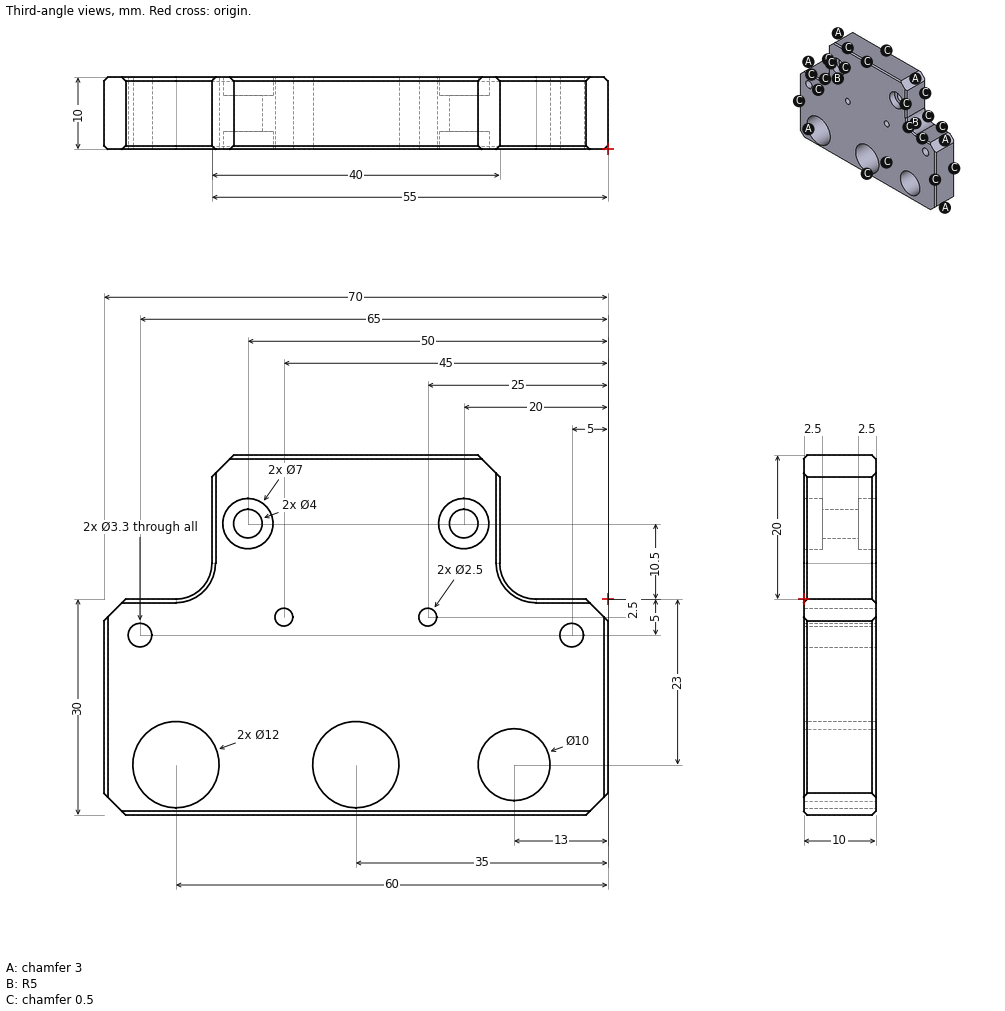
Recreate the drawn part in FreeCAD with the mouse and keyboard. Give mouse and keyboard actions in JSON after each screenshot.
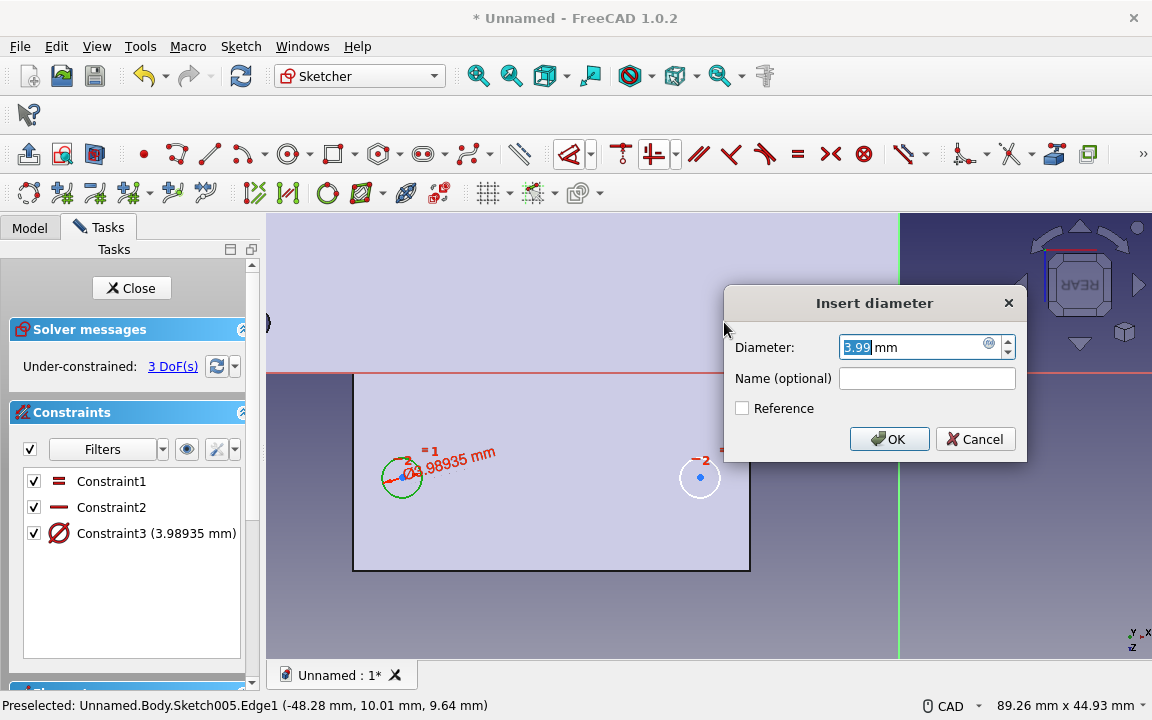
{"action": "type", "text": "4"}
{"action": "key", "text": "Return"}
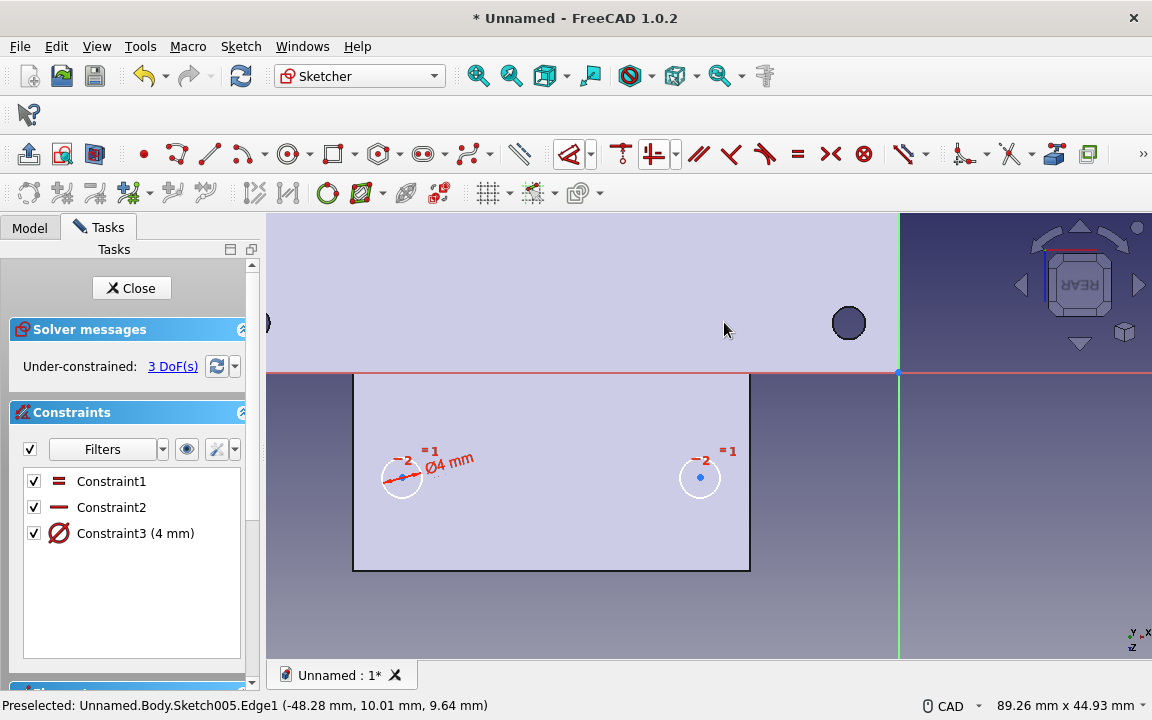
{"action": "left_click", "coordinate": [402, 478]}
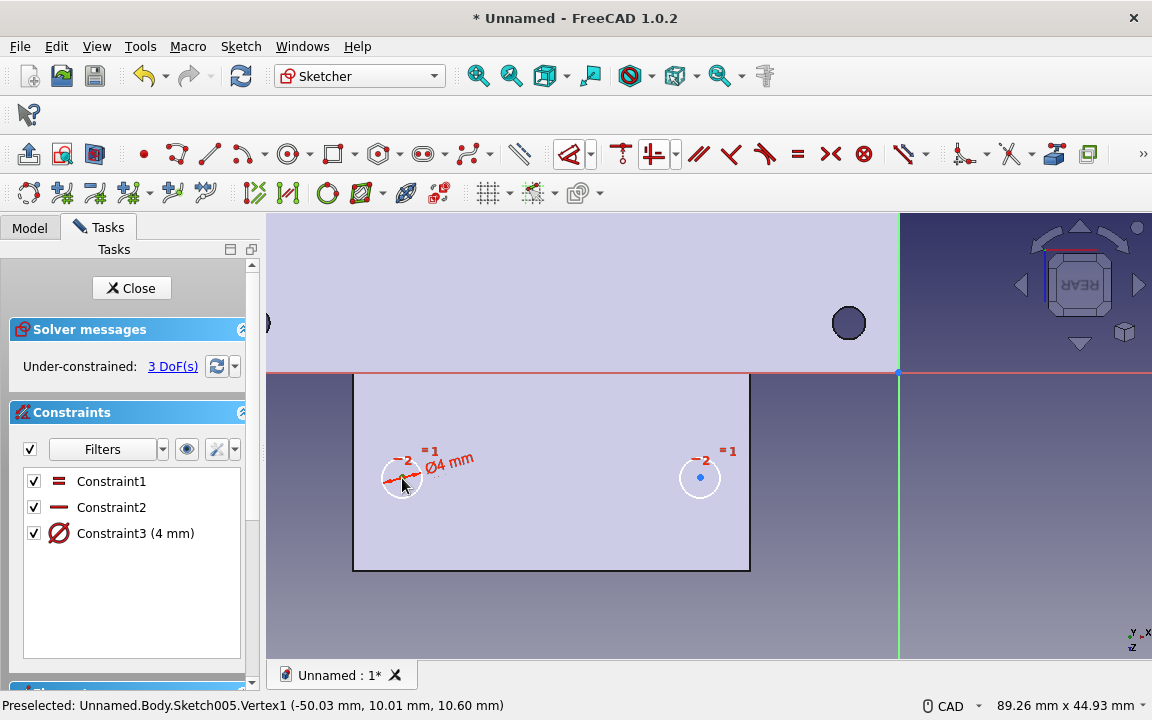
{"action": "left_click", "coordinate": [590, 154]}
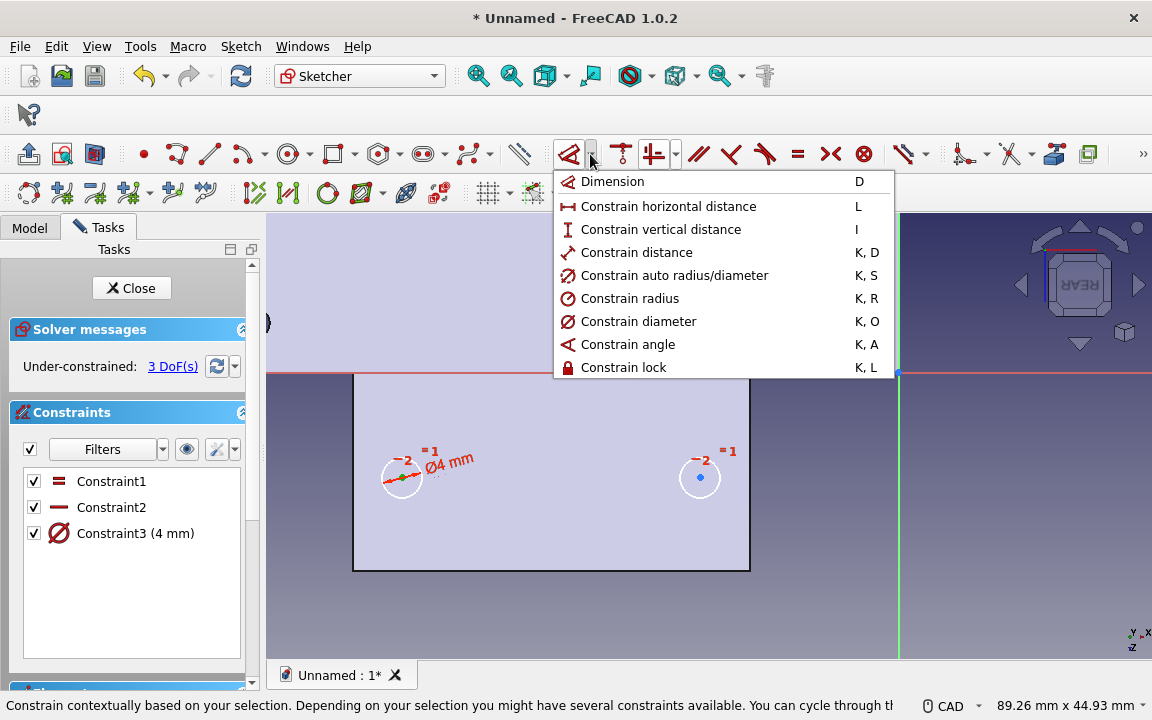
{"action": "left_click", "coordinate": [724, 206]}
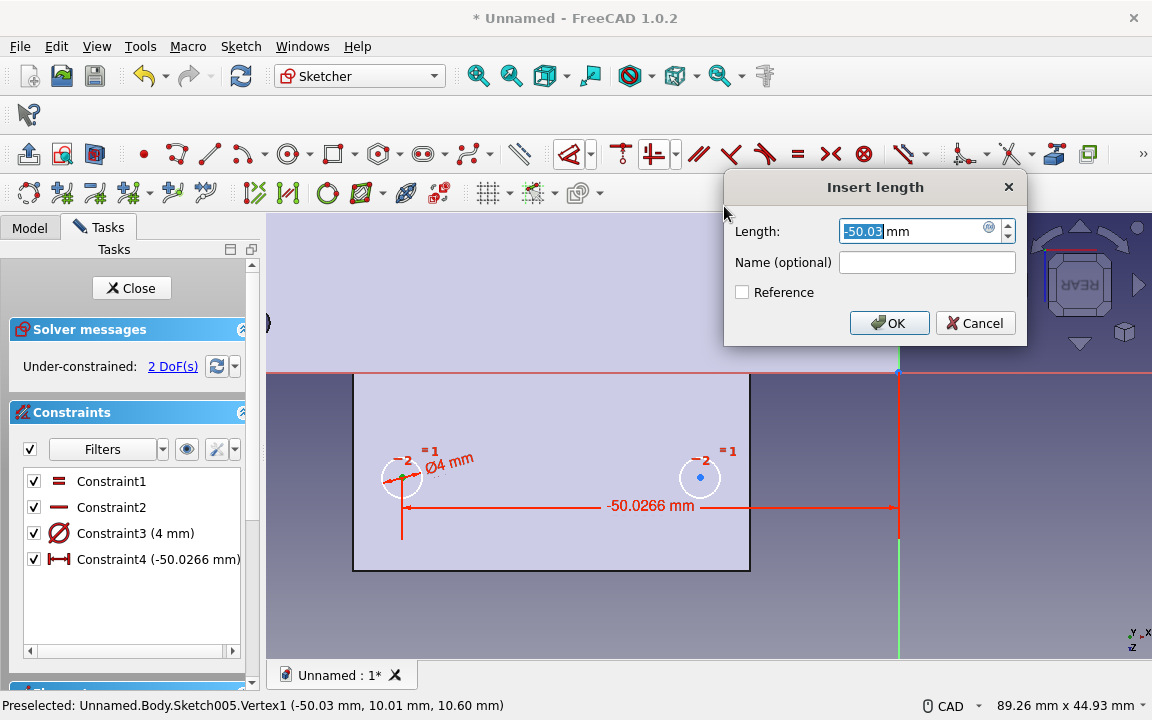
{"action": "type", "text": "-50"}
{"action": "key", "text": "Return"}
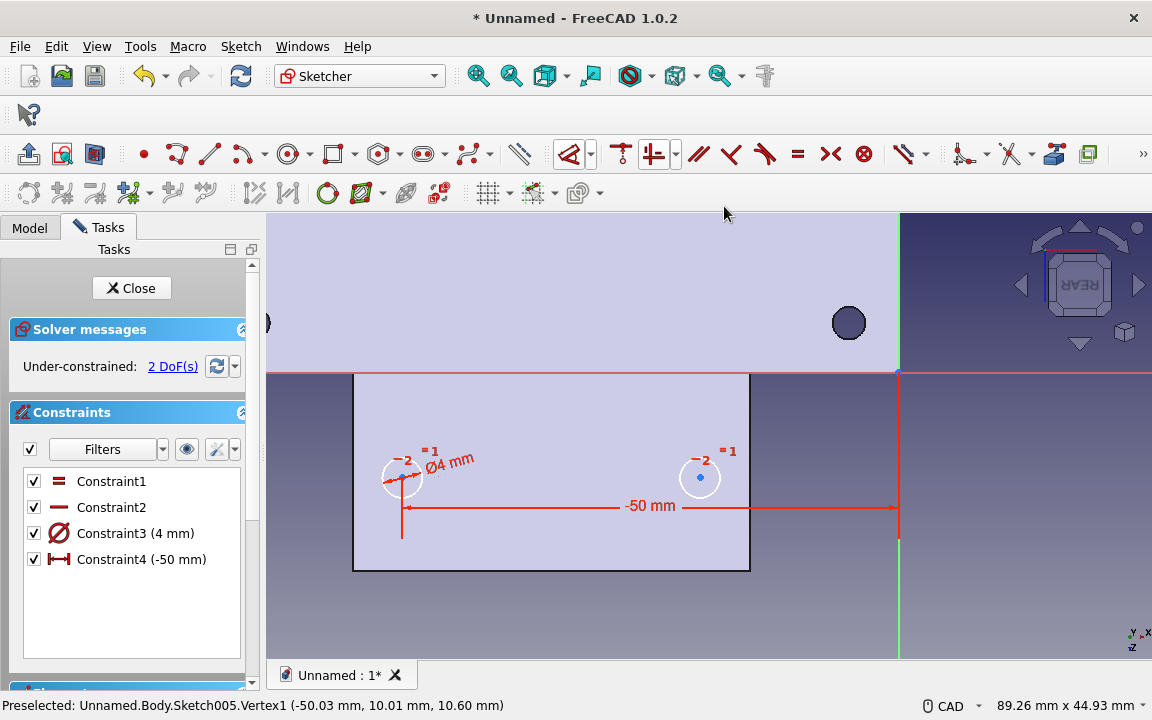
{"action": "left_click", "coordinate": [700, 478]}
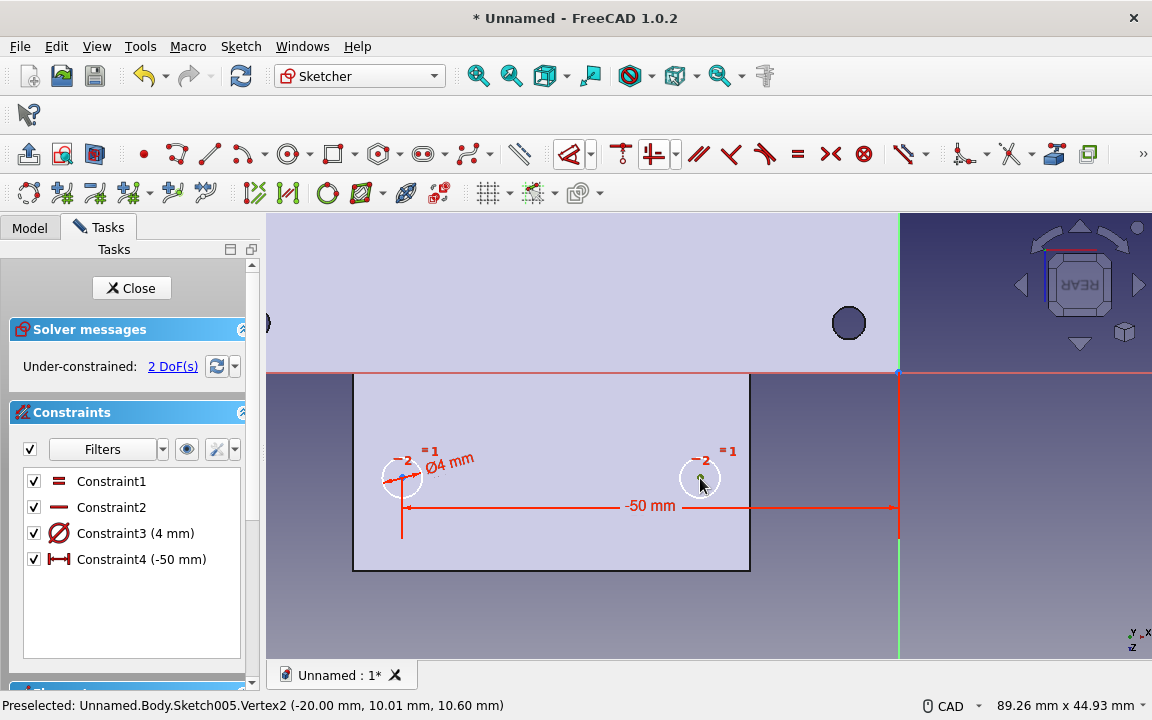
{"action": "key", "text": "l"}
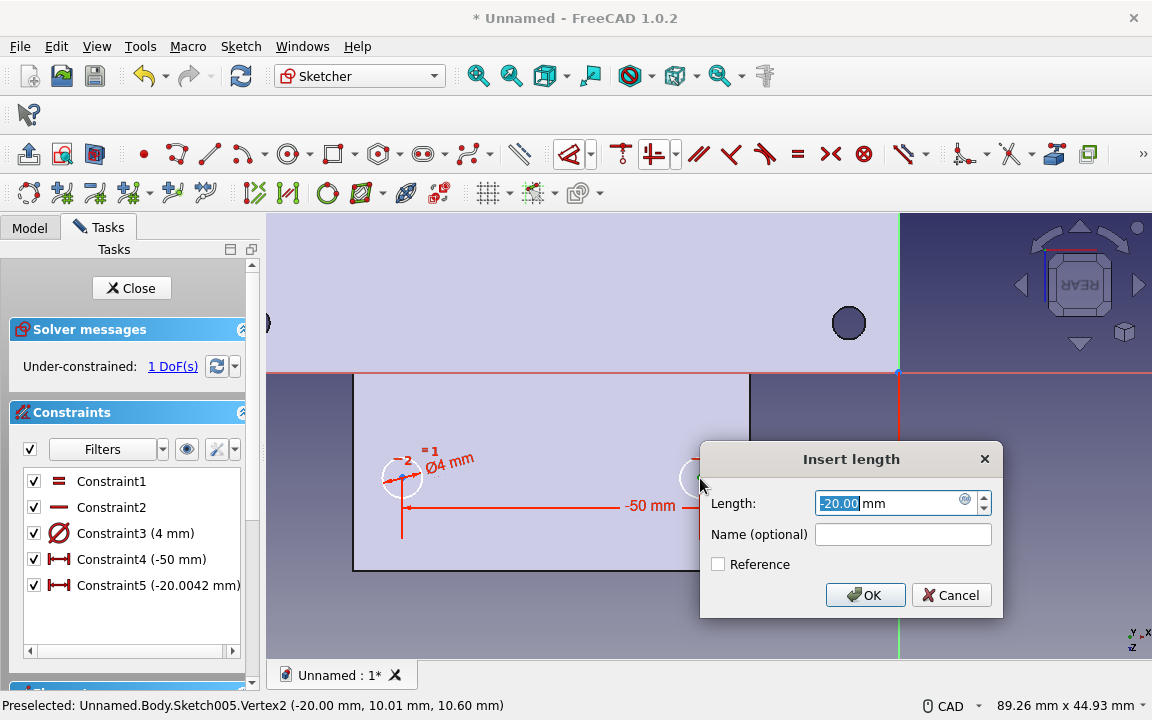
{"action": "type", "text": "-20"}
{"action": "key", "text": "Return"}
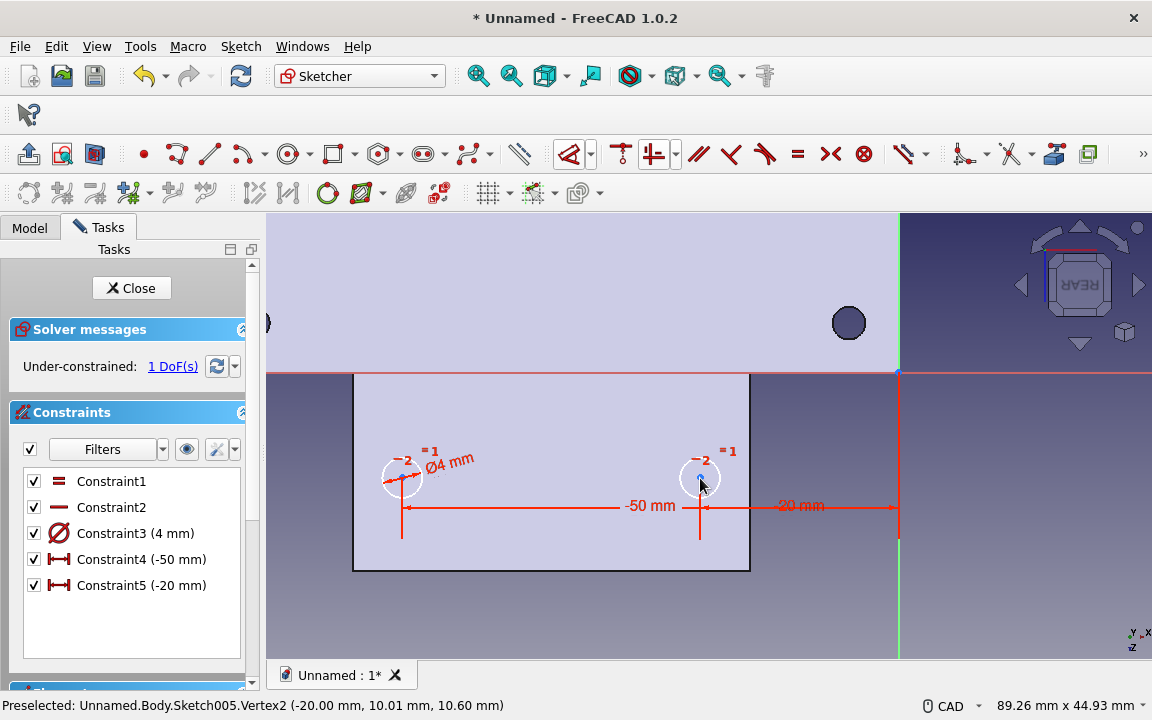
{"action": "left_click", "coordinate": [402, 478]}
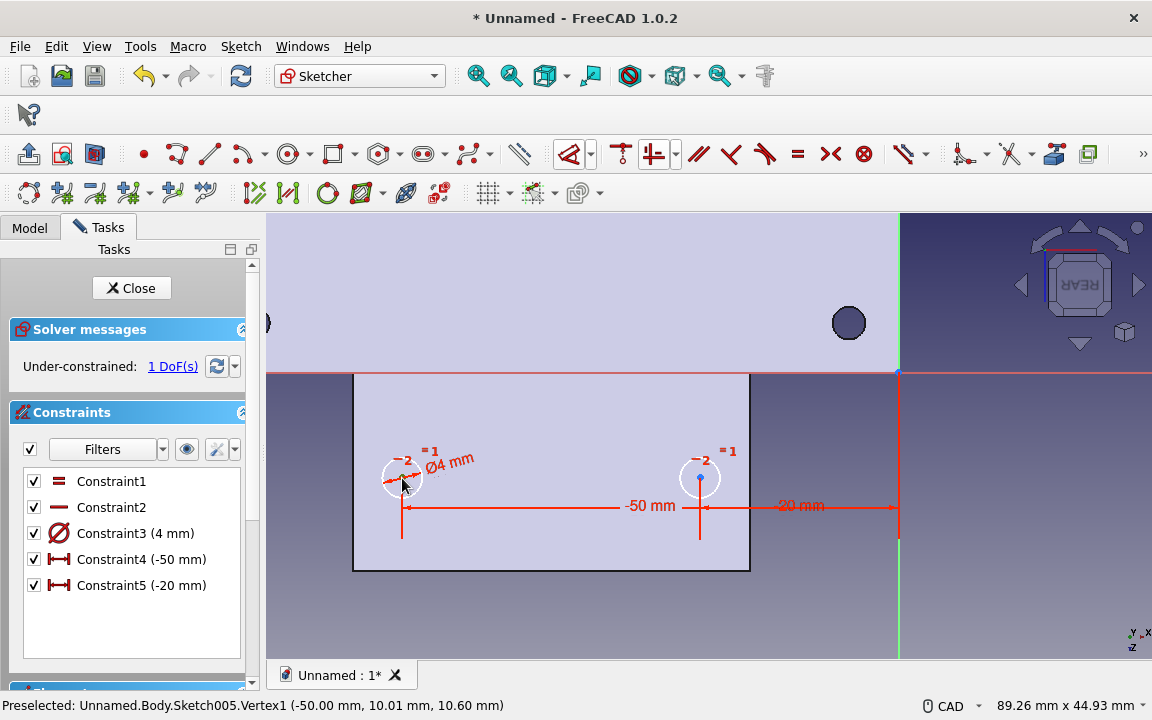
{"action": "left_click", "coordinate": [590, 154]}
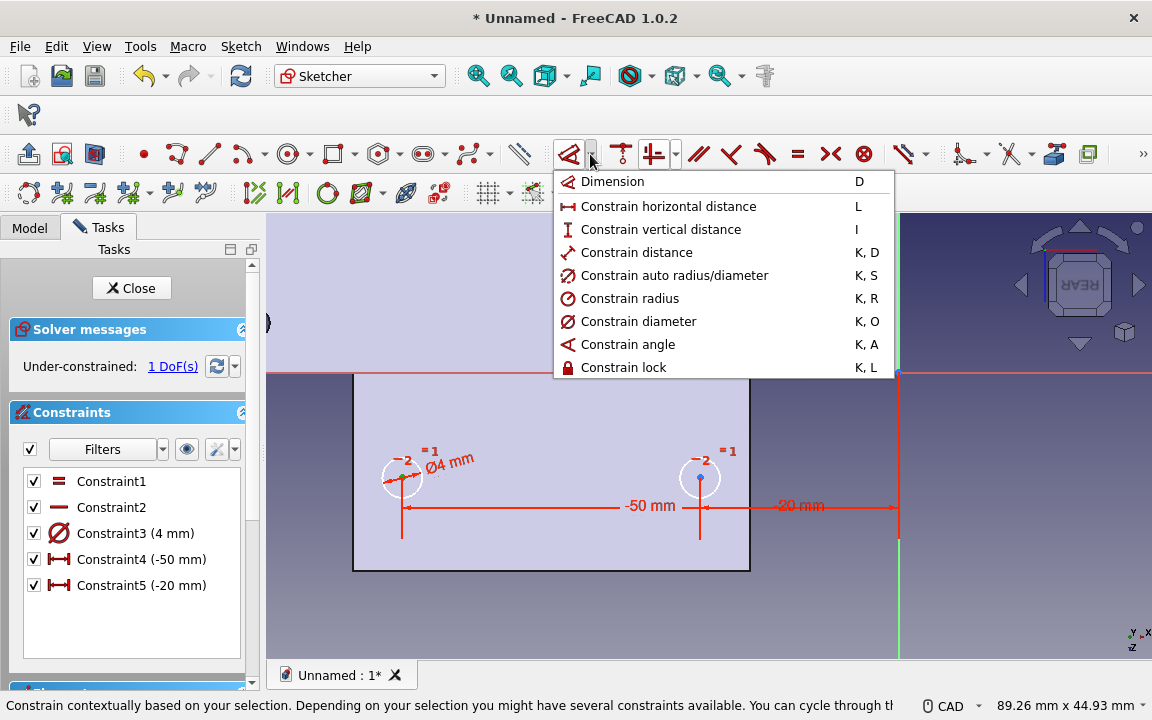
{"action": "left_click", "coordinate": [724, 230]}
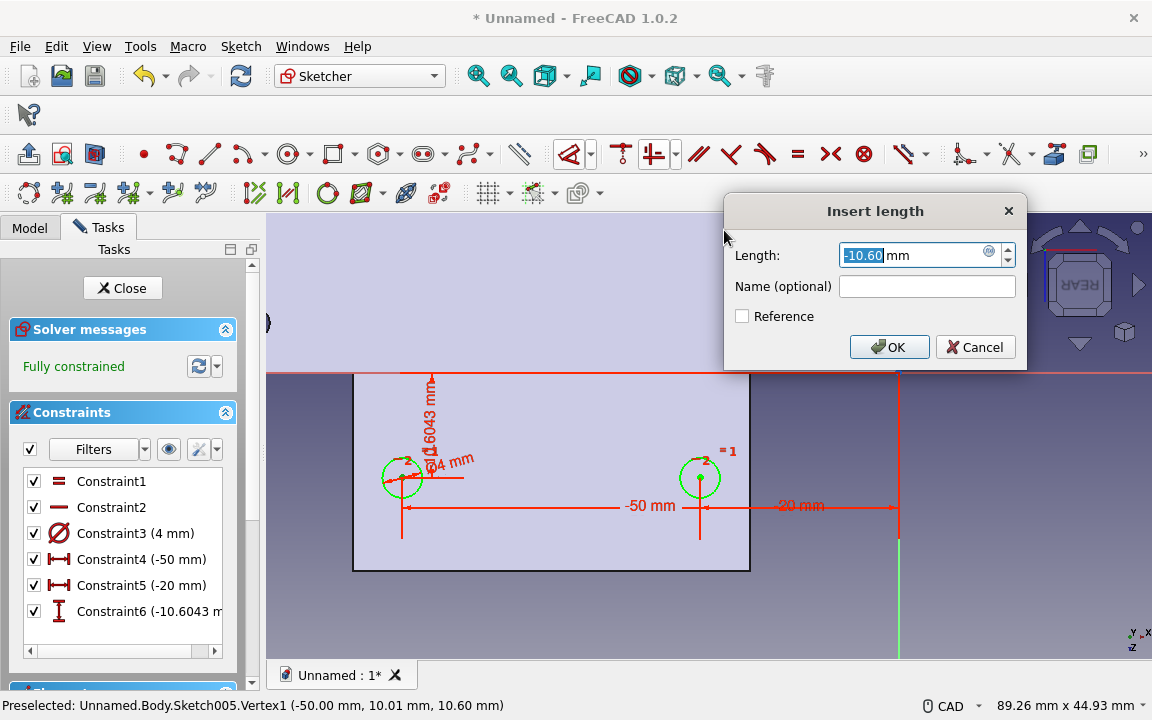
{"action": "type", "text": "-10.5"}
{"action": "key", "text": "Return"}